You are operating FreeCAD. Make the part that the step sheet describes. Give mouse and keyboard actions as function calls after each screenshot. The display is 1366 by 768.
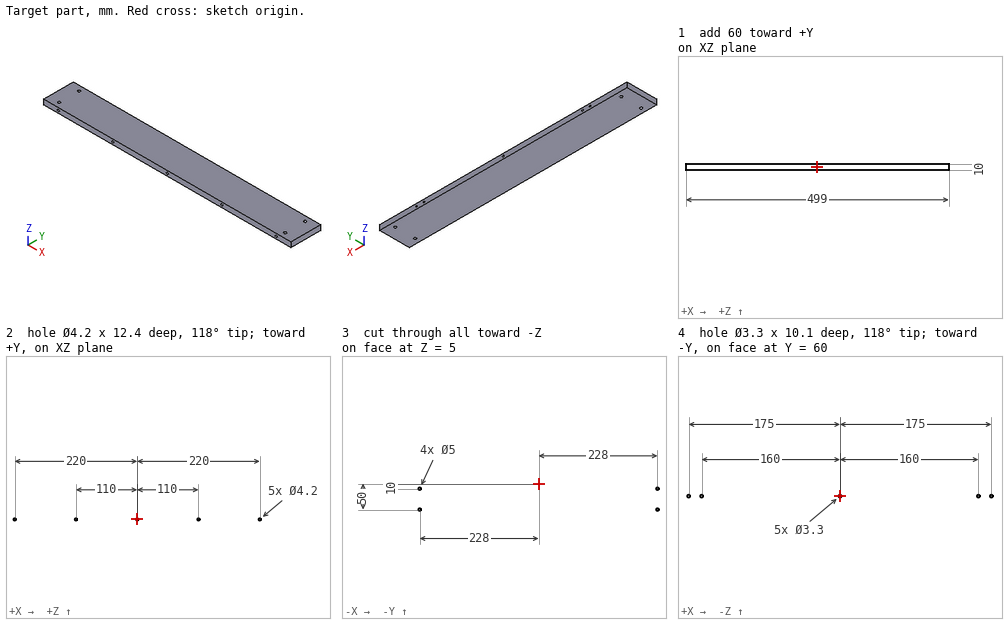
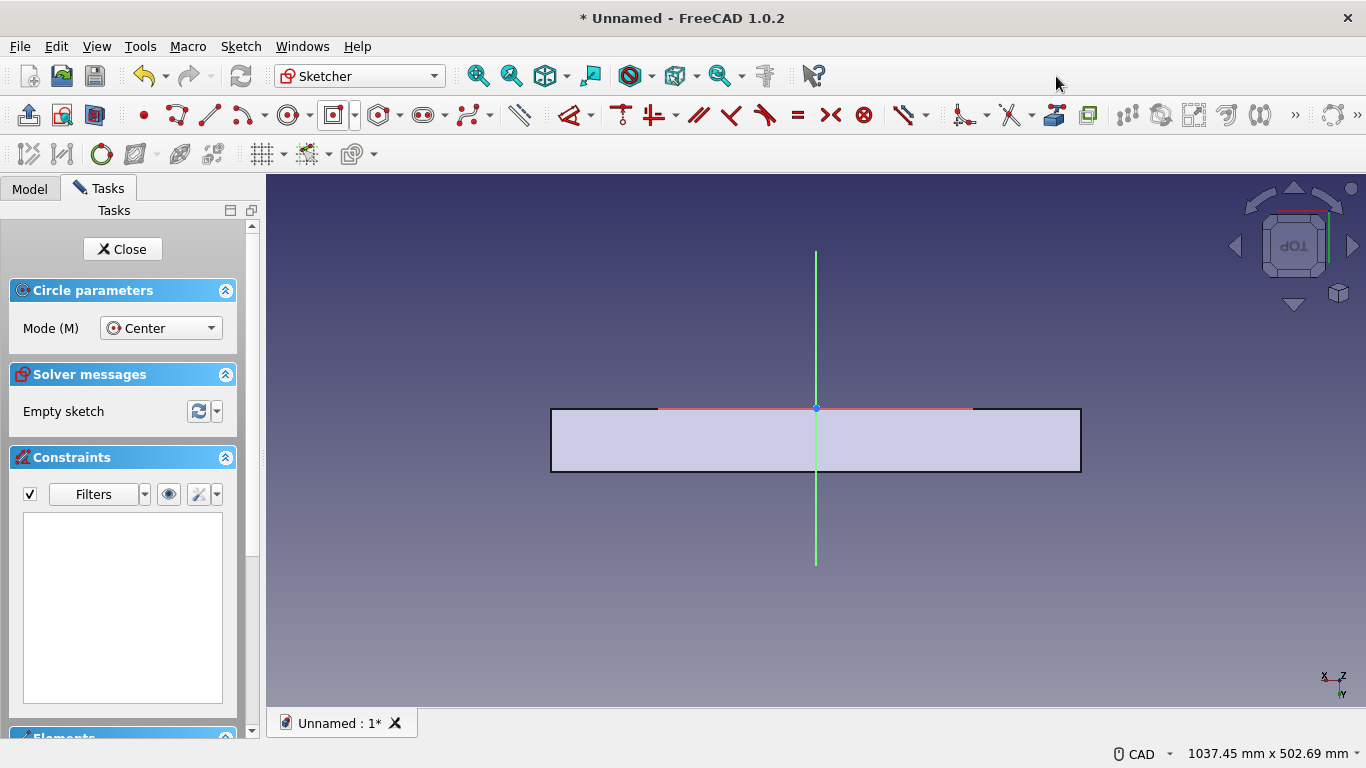
scroll(574, 462, up, 11)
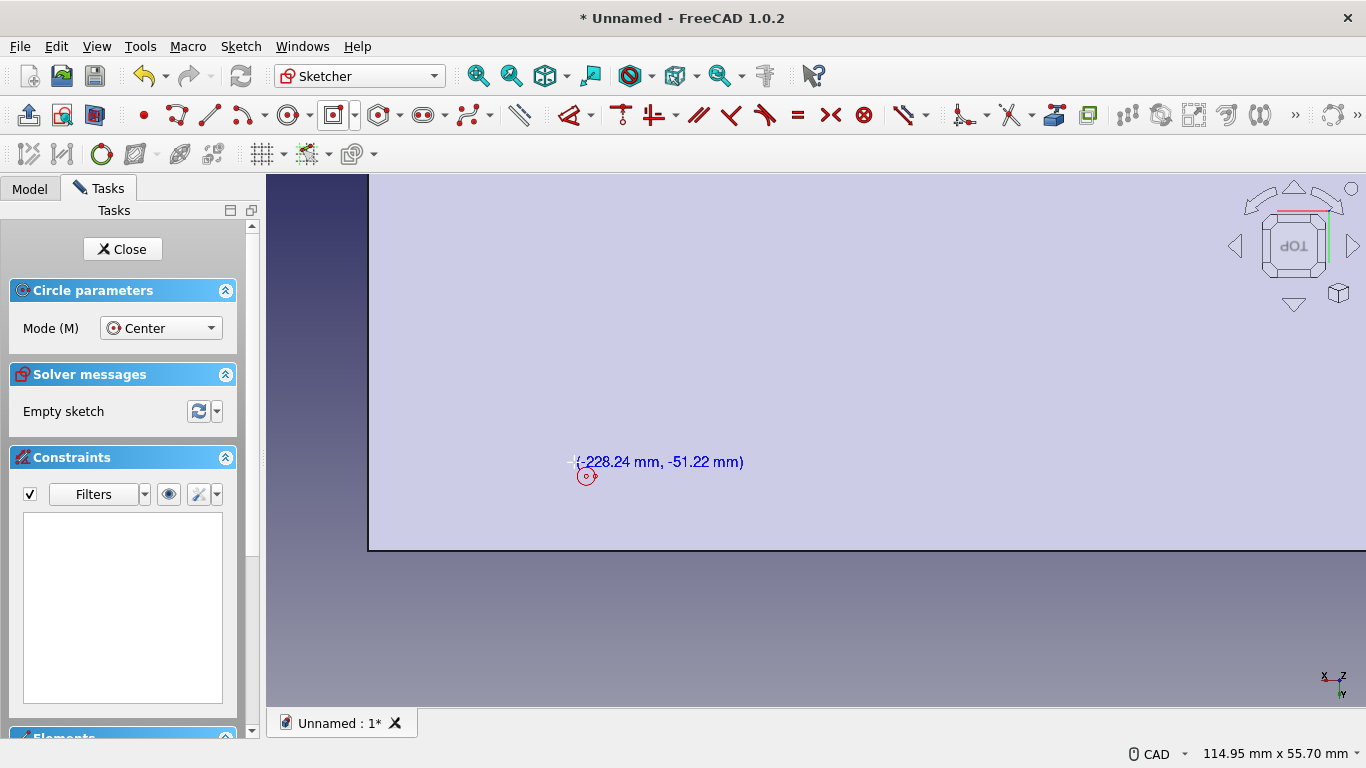
scroll(433, 474, down, 10)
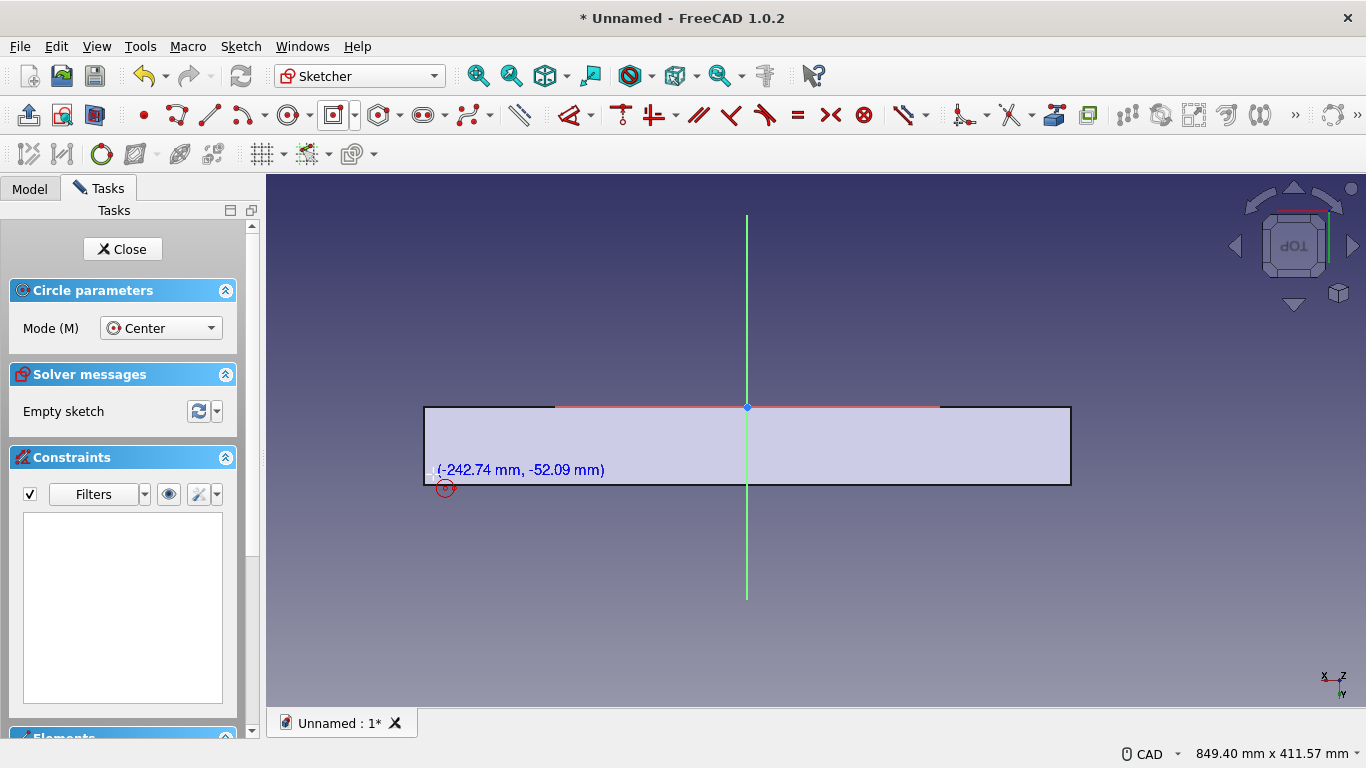
click(452, 472)
move(455, 470)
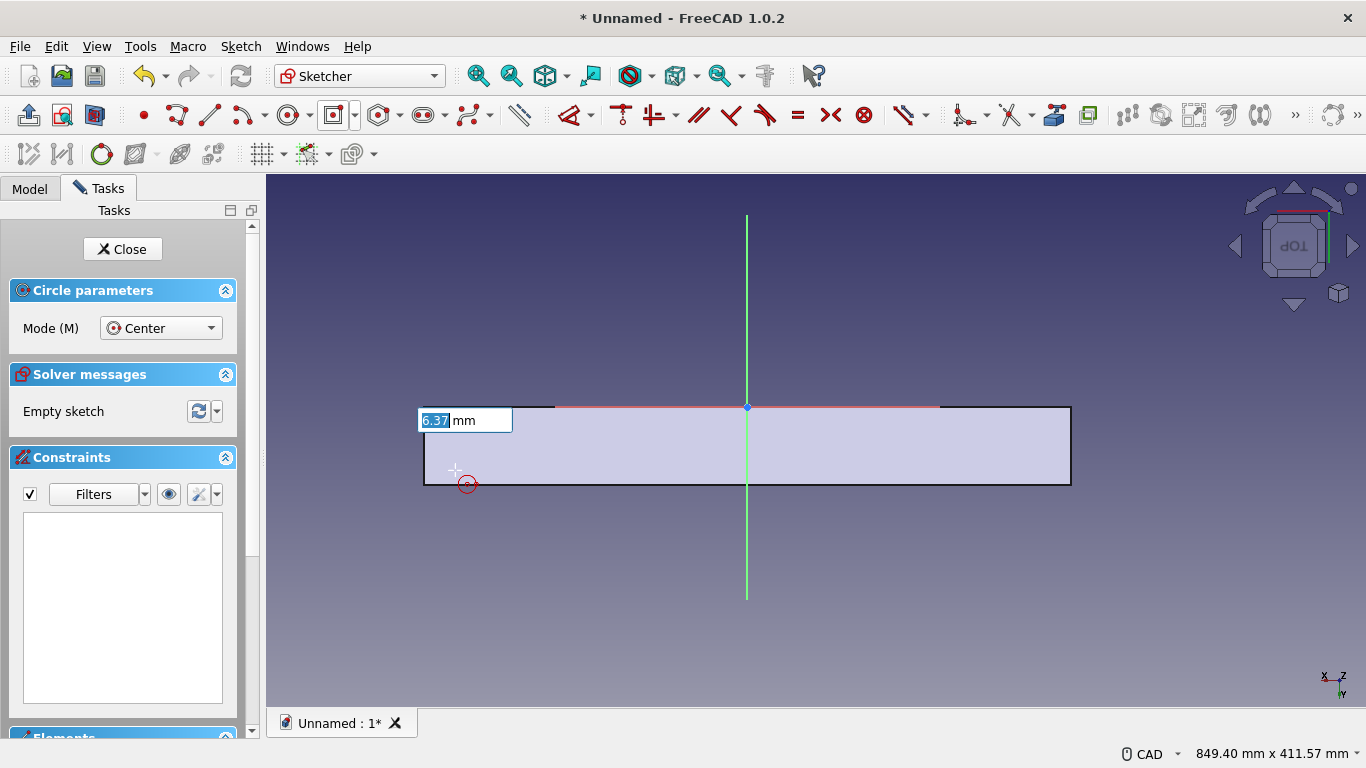
text(5)
key(Return)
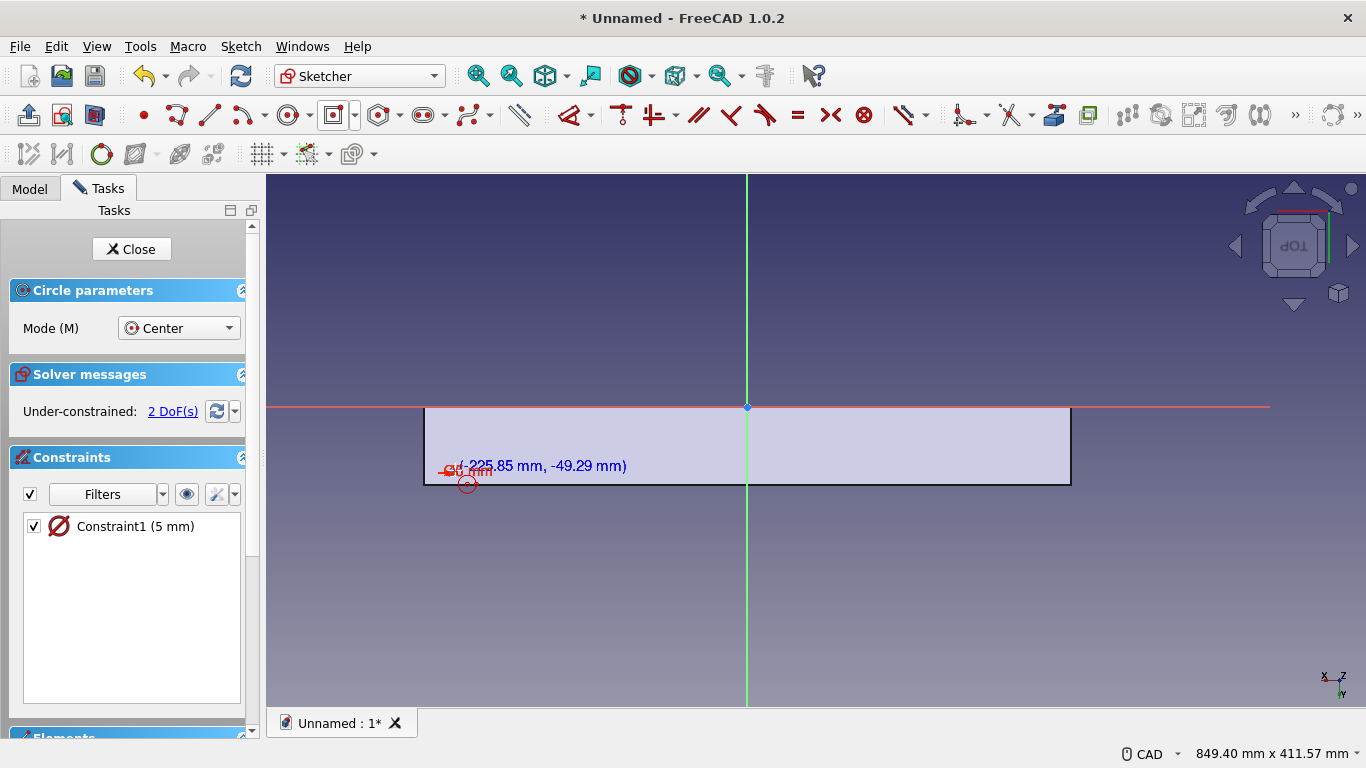
scroll(452, 420, up, 10)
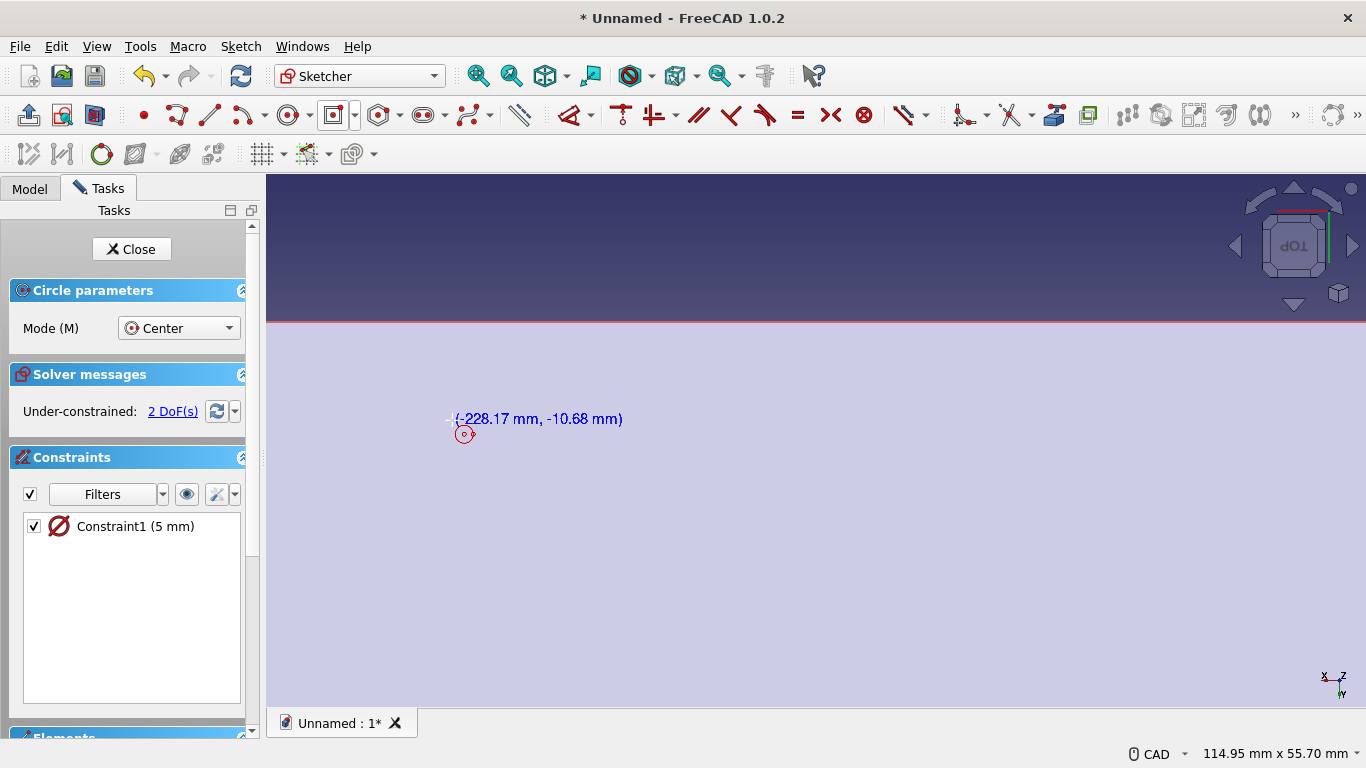
scroll(452, 420, down, 10)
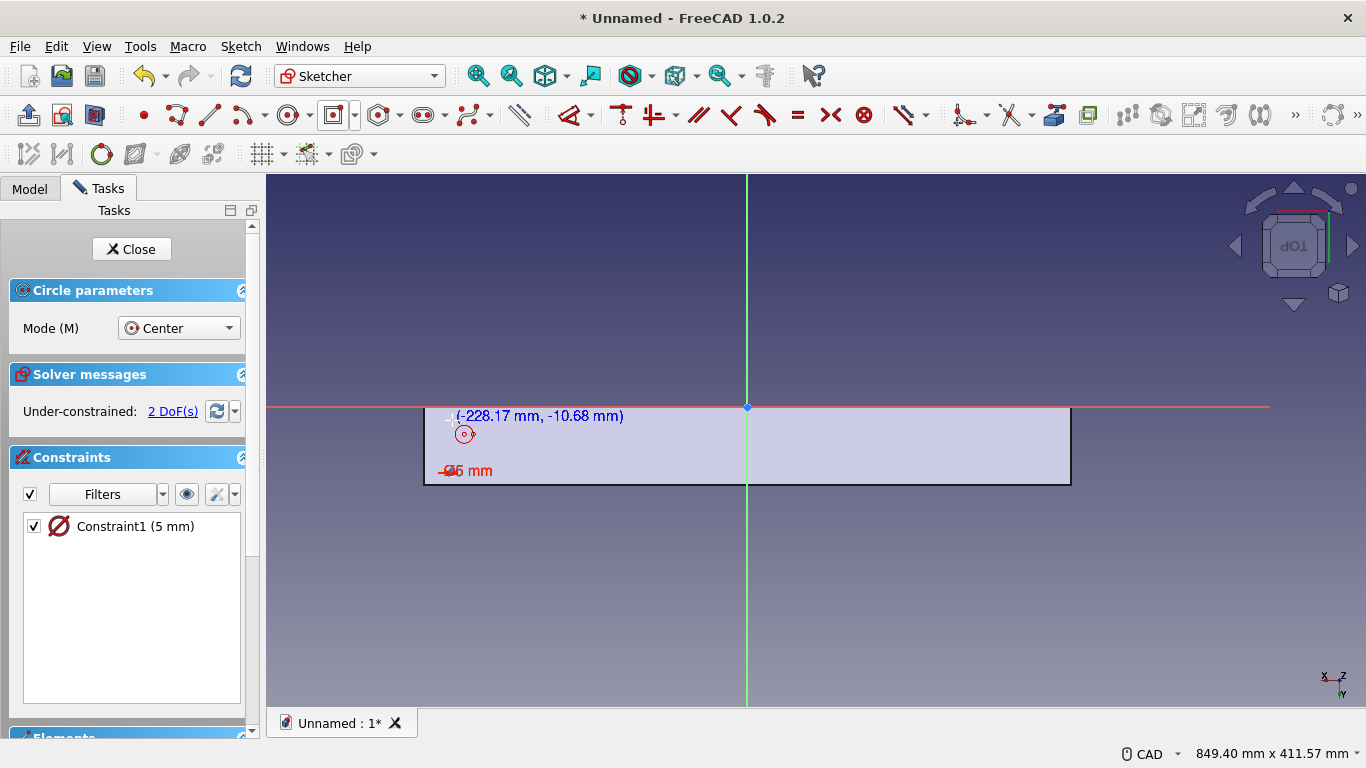
scroll(452, 420, up, 2)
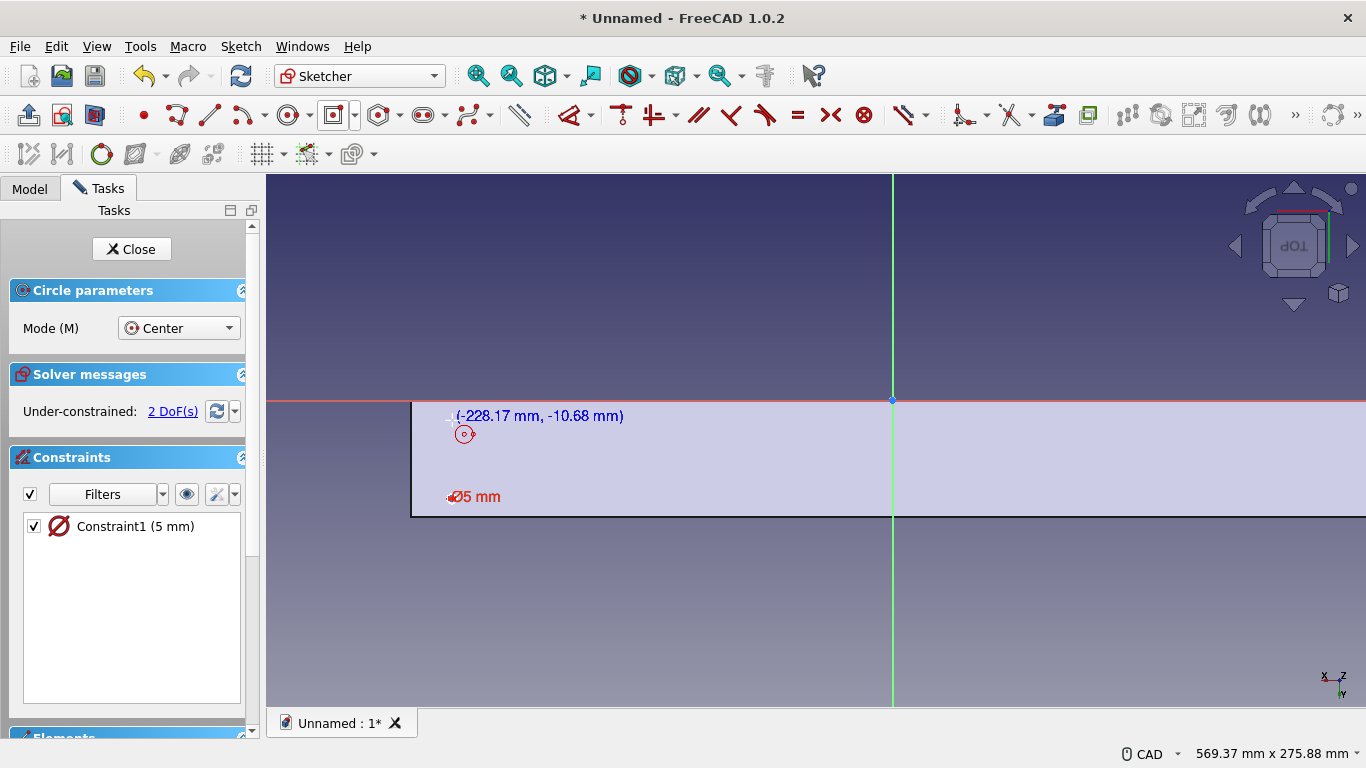
click(452, 420)
move(456, 417)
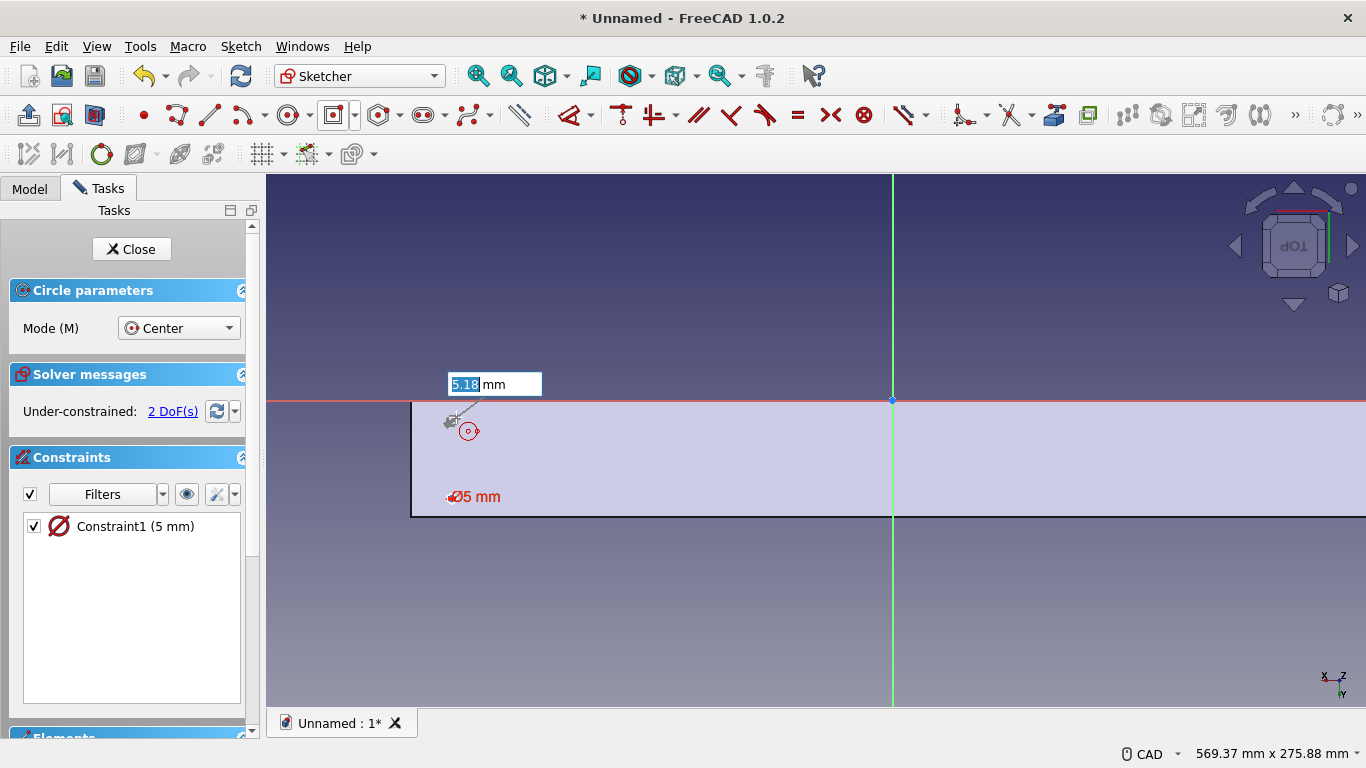
text(5)
key(Return)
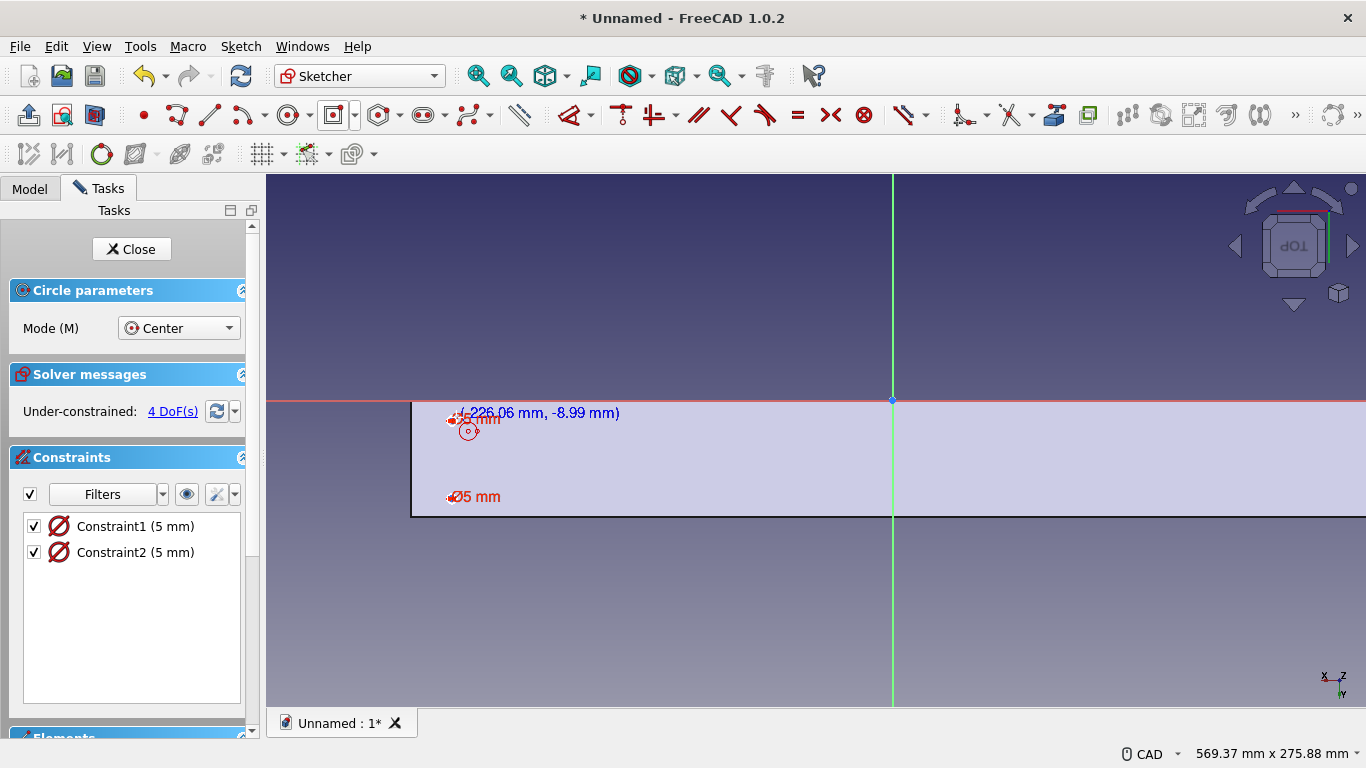
scroll(452, 418, down, 2)